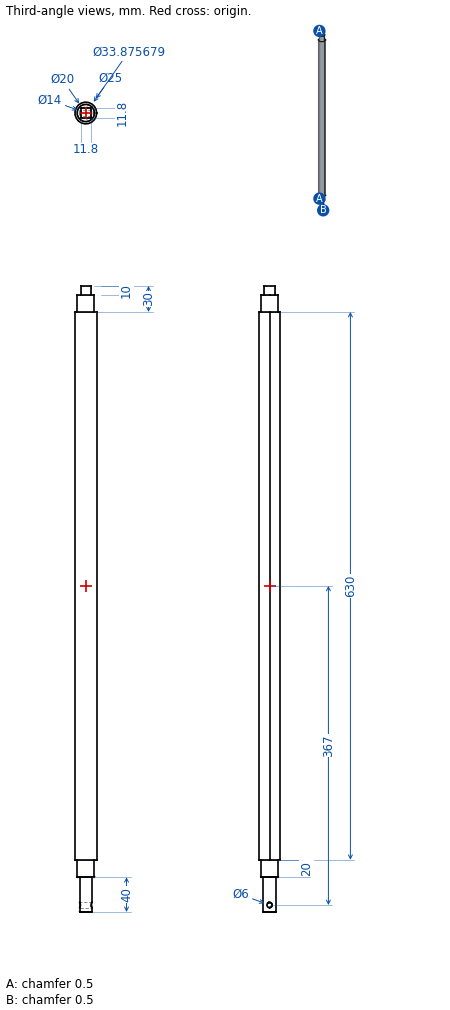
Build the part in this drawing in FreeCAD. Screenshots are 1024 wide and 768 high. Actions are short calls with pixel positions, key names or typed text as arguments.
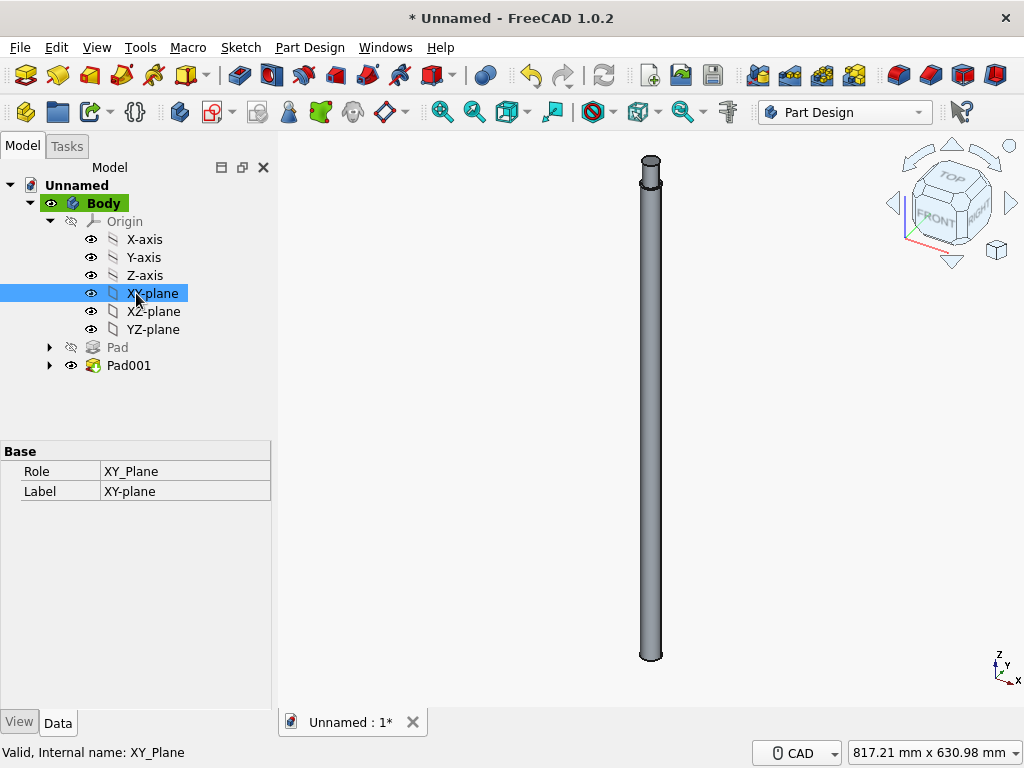
click(386, 112)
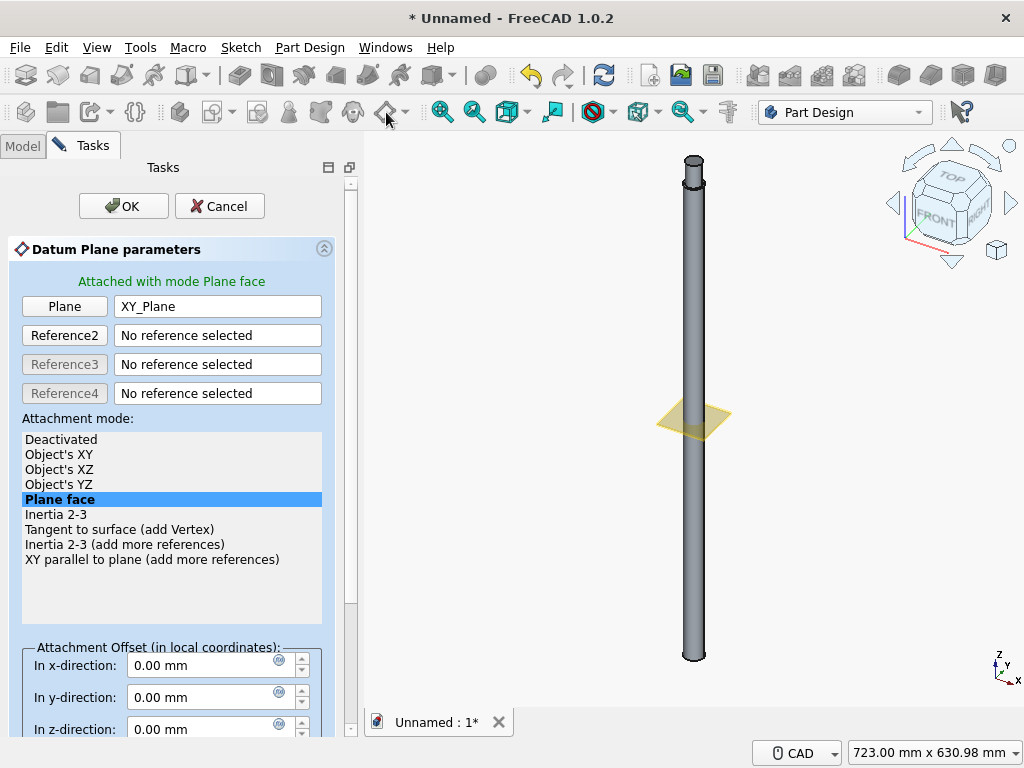
scroll(351, 456, down, 2)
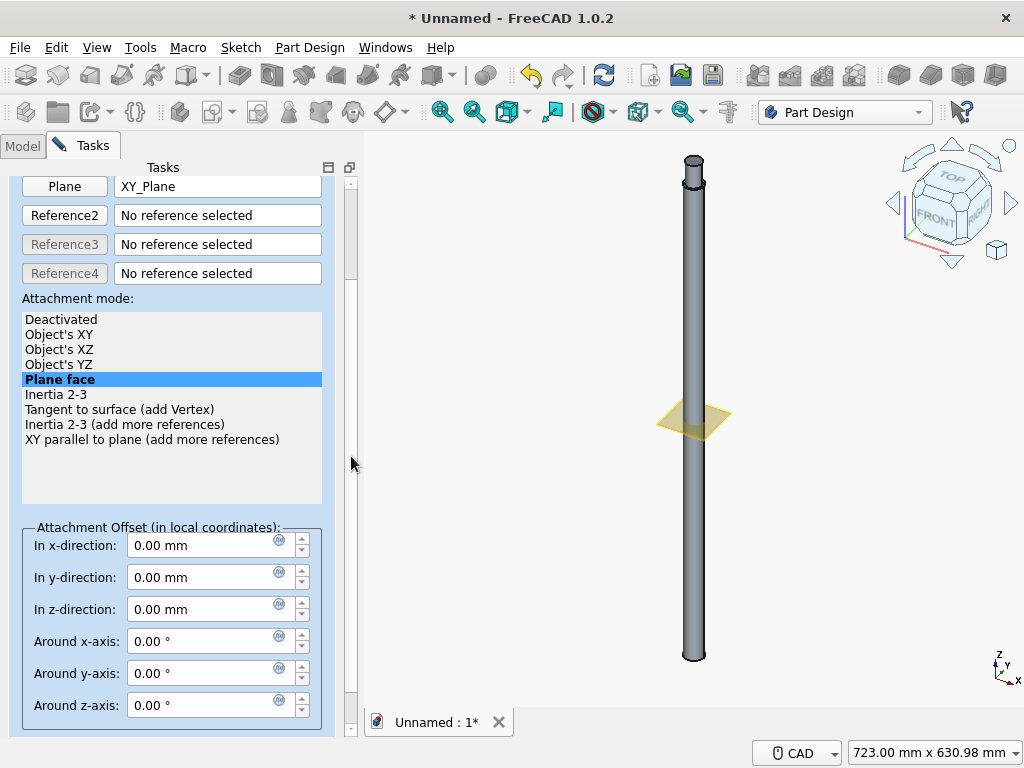
triple_click(210, 609)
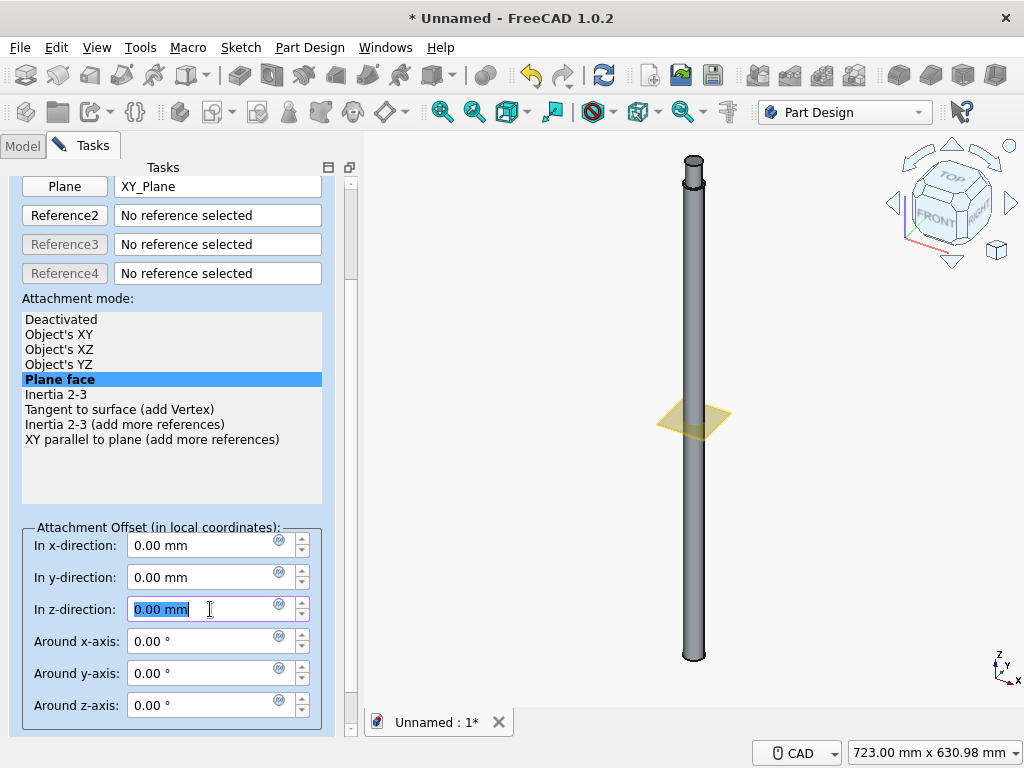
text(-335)
key(Tab)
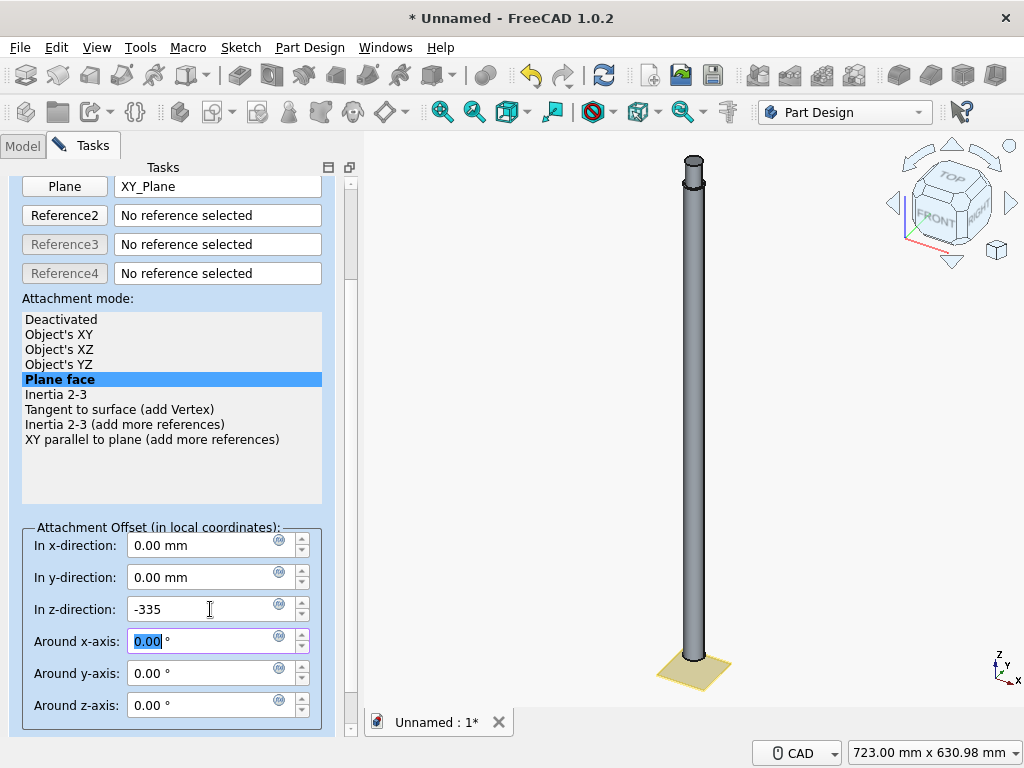
scroll(351, 456, up, 3)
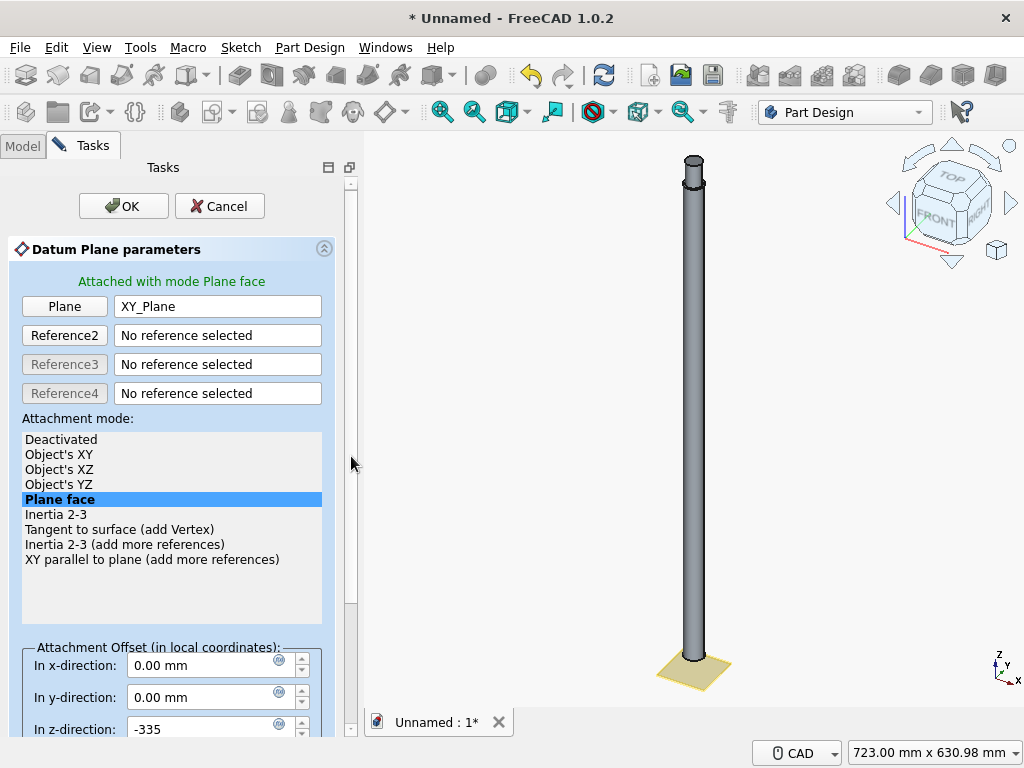
click(124, 206)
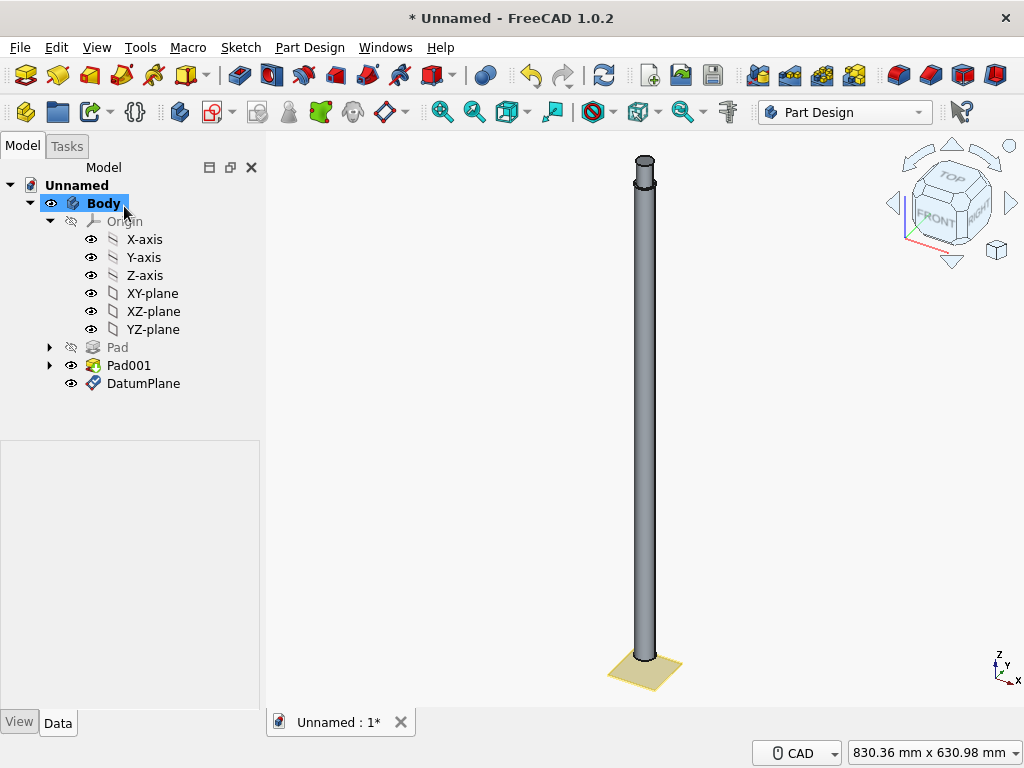
click(116, 383)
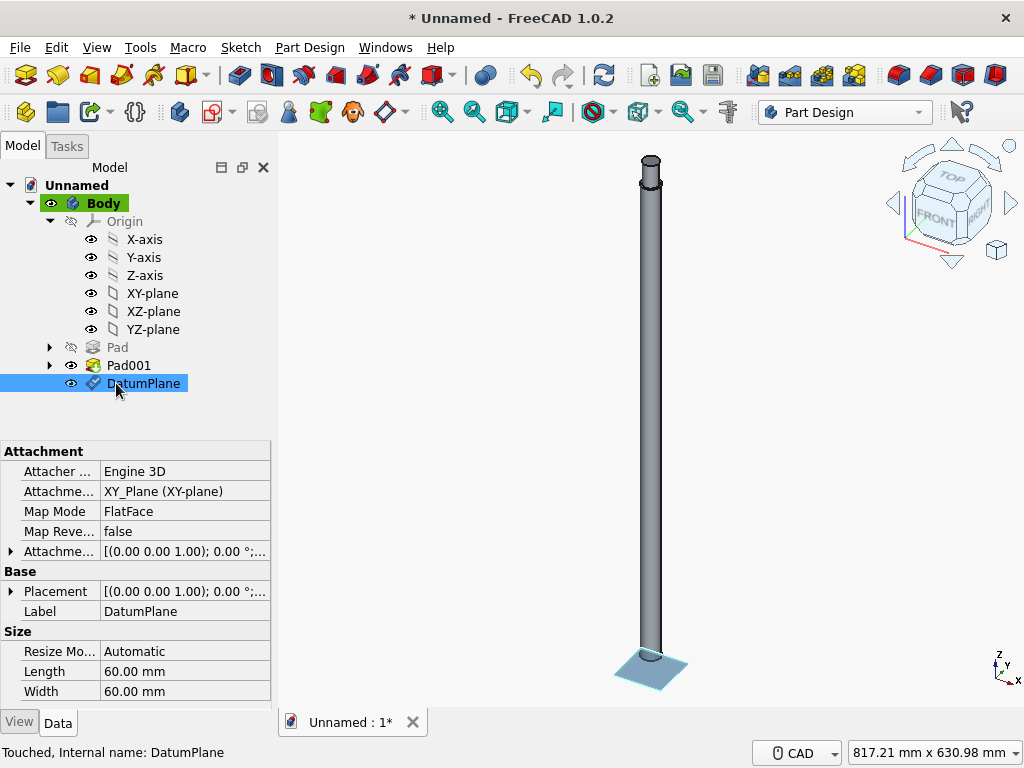
click(212, 112)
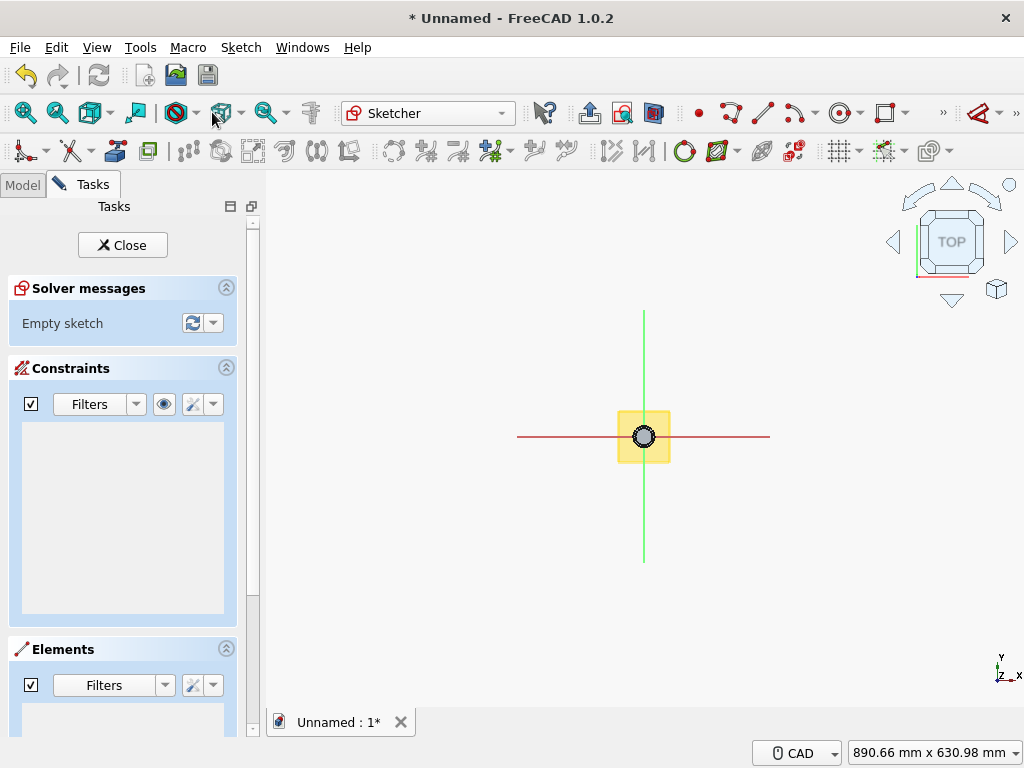
click(654, 114)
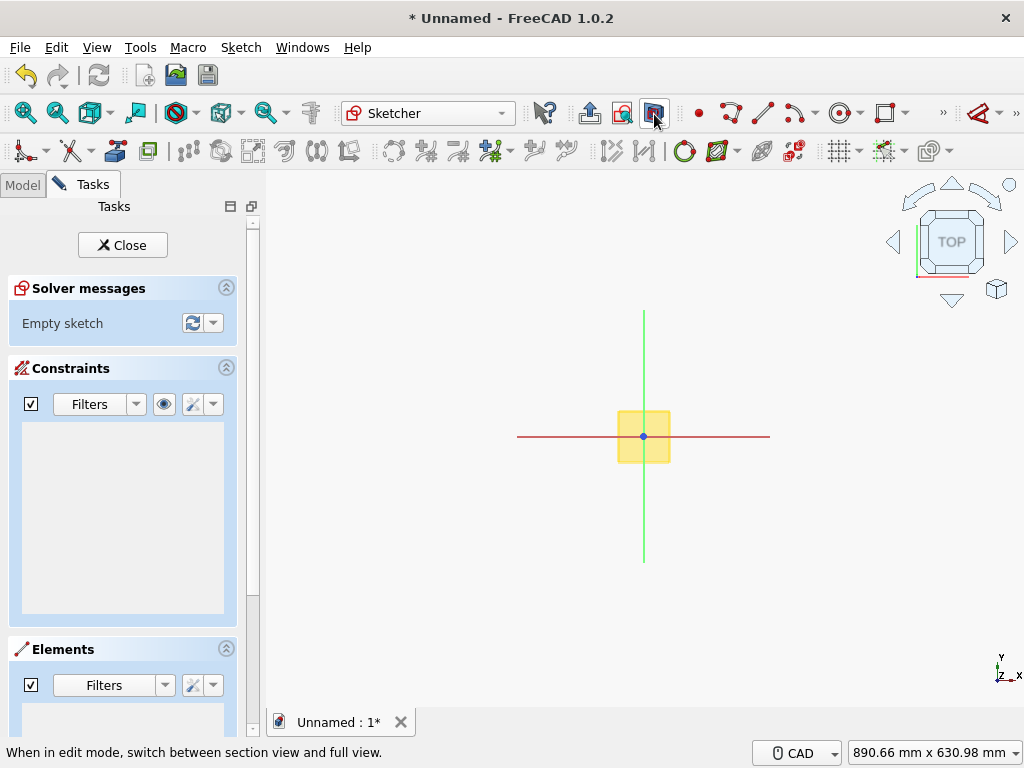
scroll(648, 437, up, 15)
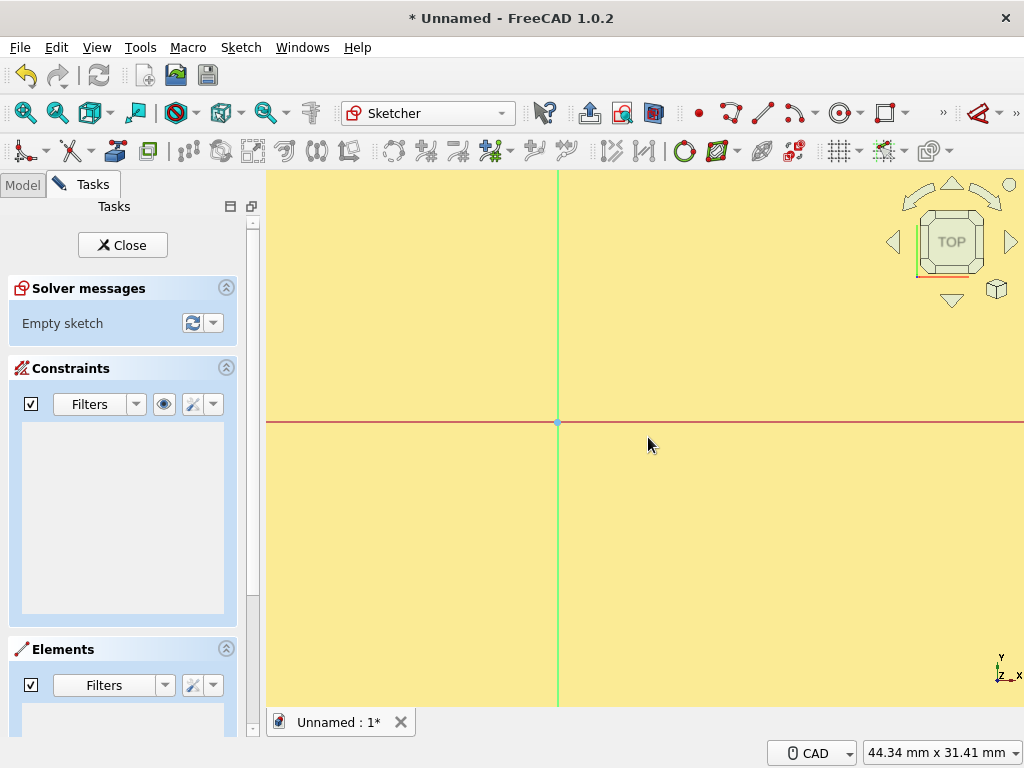
click(840, 114)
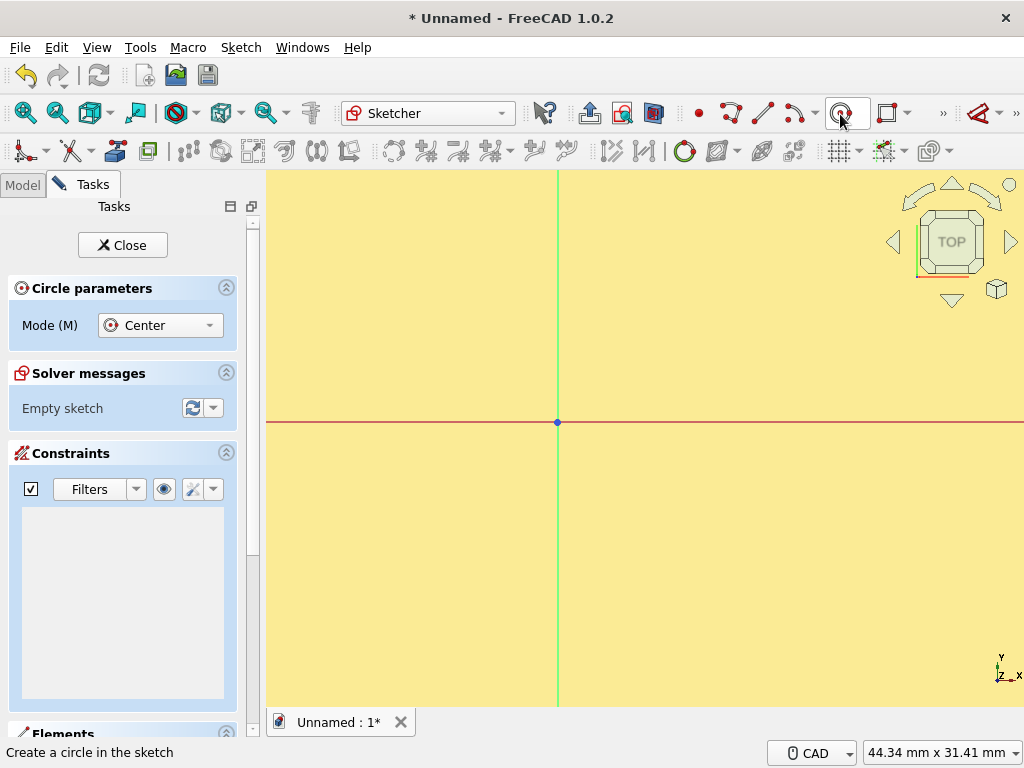
click(558, 422)
move(679, 301)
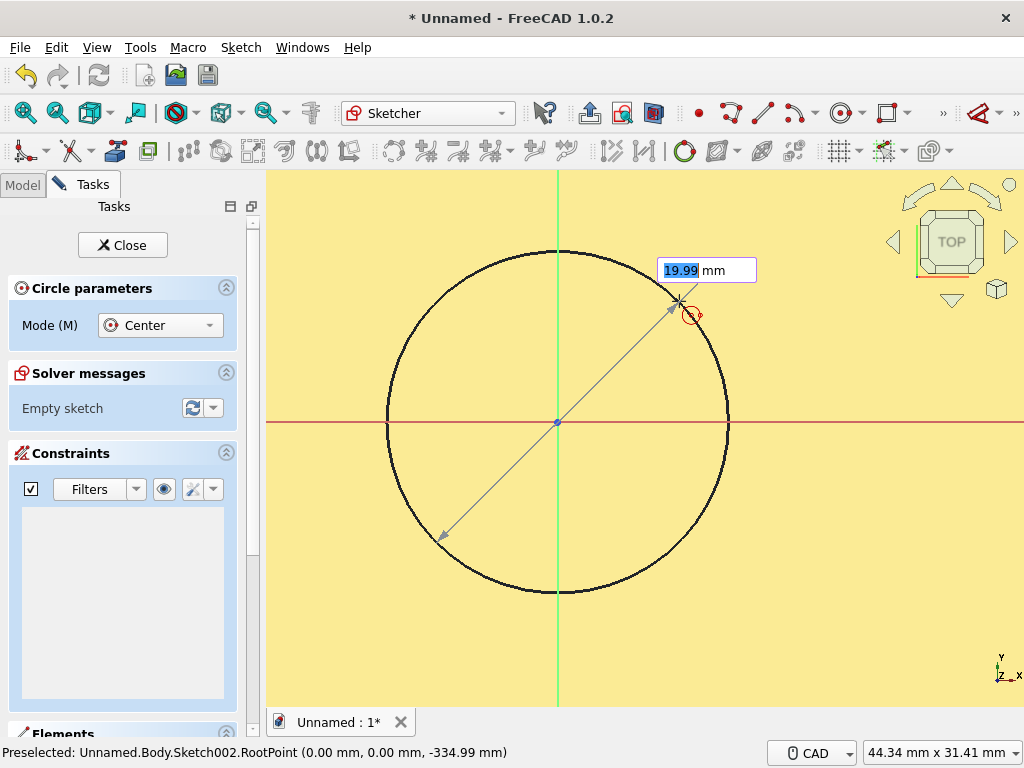
text(20)
key(Return)
key(Escape)